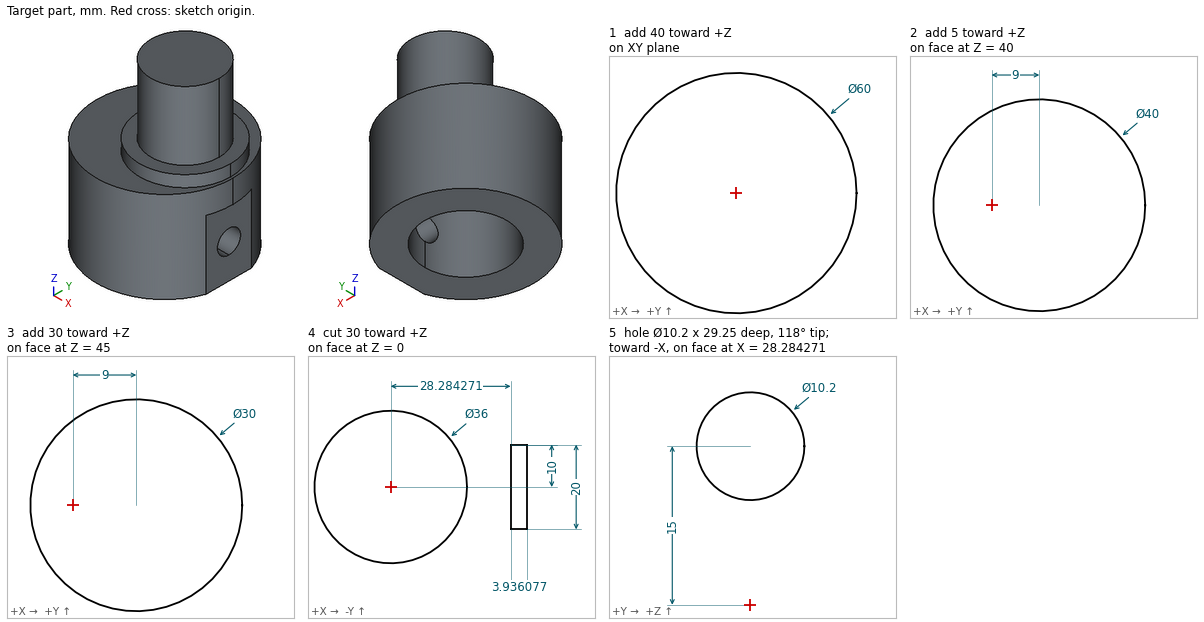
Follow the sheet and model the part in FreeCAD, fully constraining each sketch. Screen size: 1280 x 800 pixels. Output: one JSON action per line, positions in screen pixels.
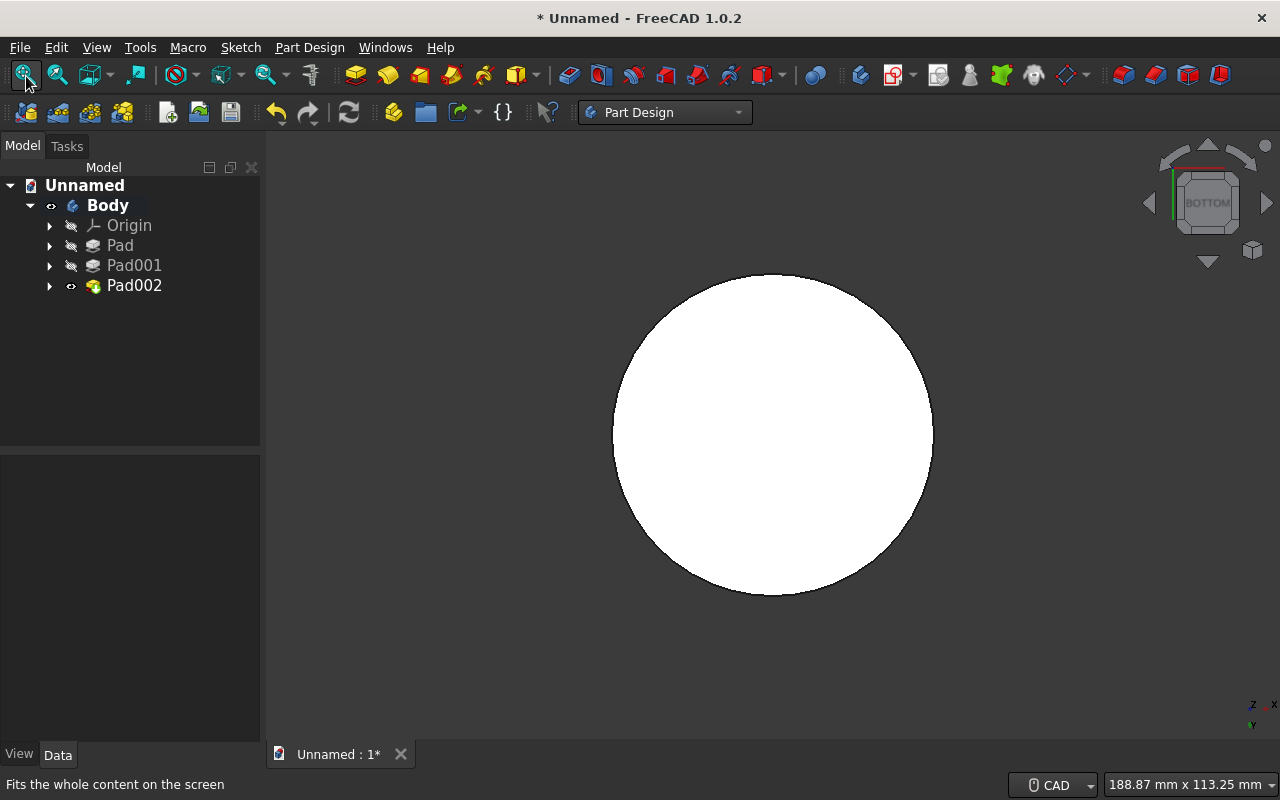
{"action": "left_click", "coordinate": [773, 434]}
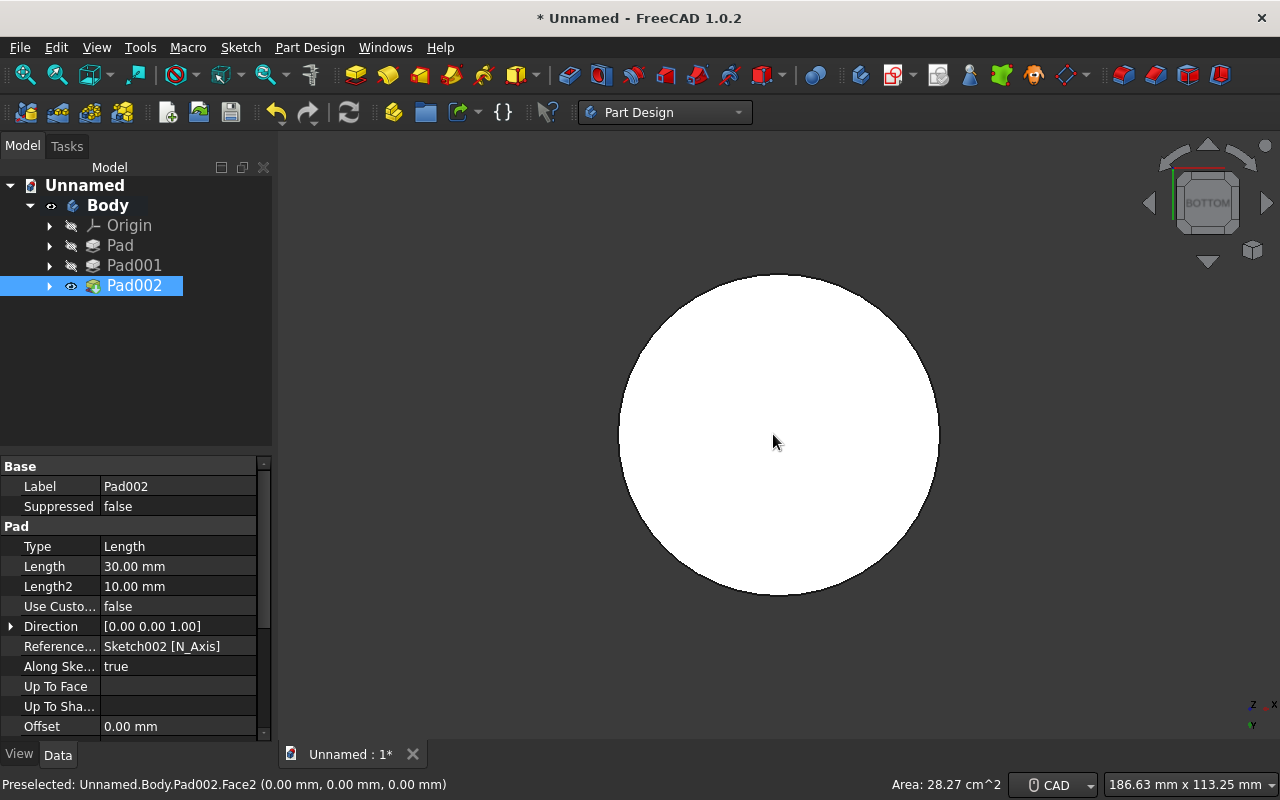
{"action": "left_click", "coordinate": [894, 76]}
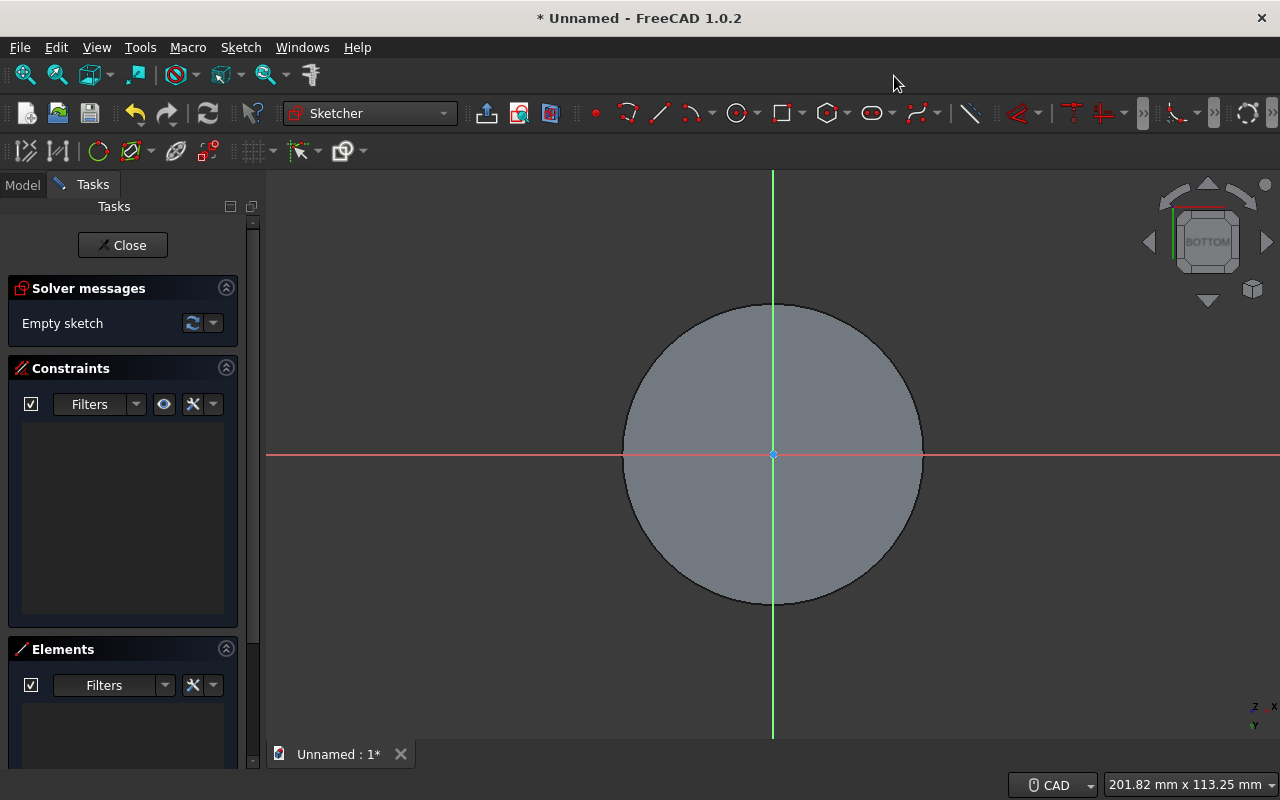
{"action": "scroll", "coordinate": [935, 454], "scroll_direction": "up", "scroll_amount": 3}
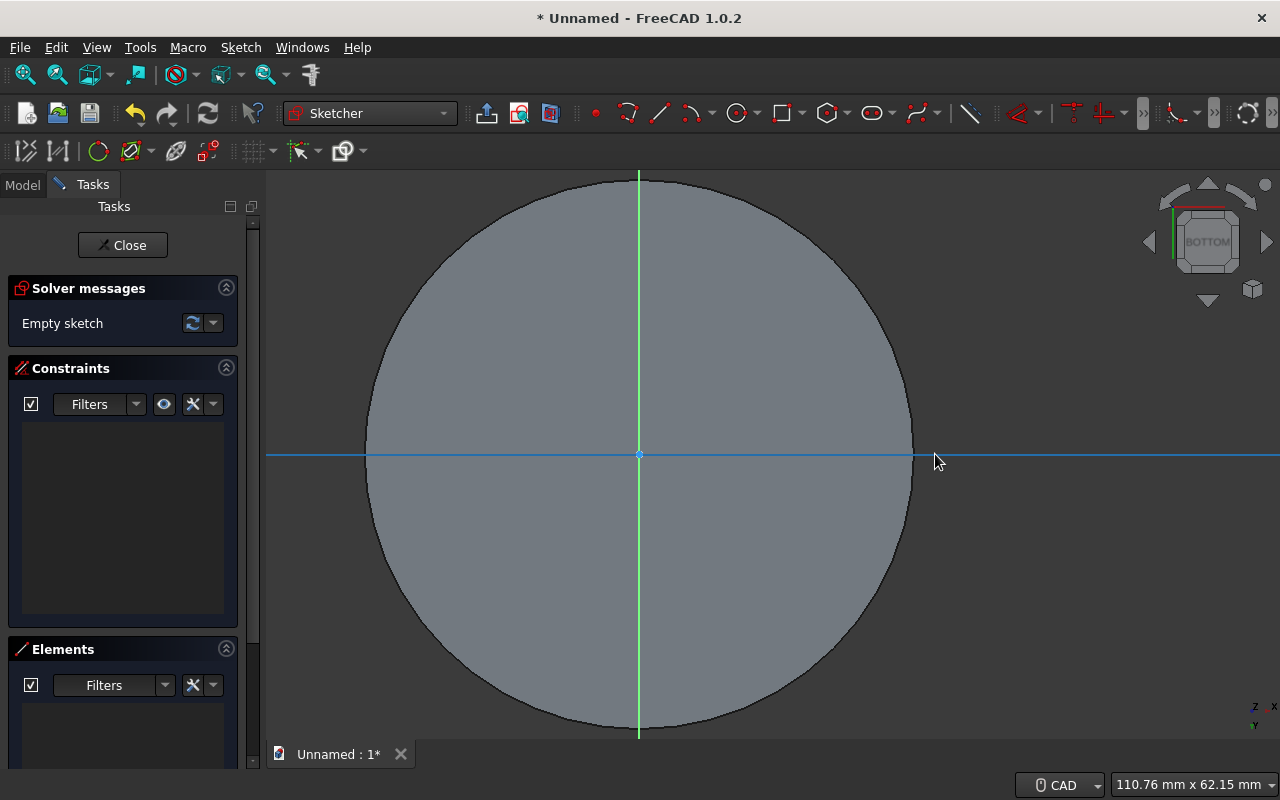
{"action": "left_click", "coordinate": [782, 114]}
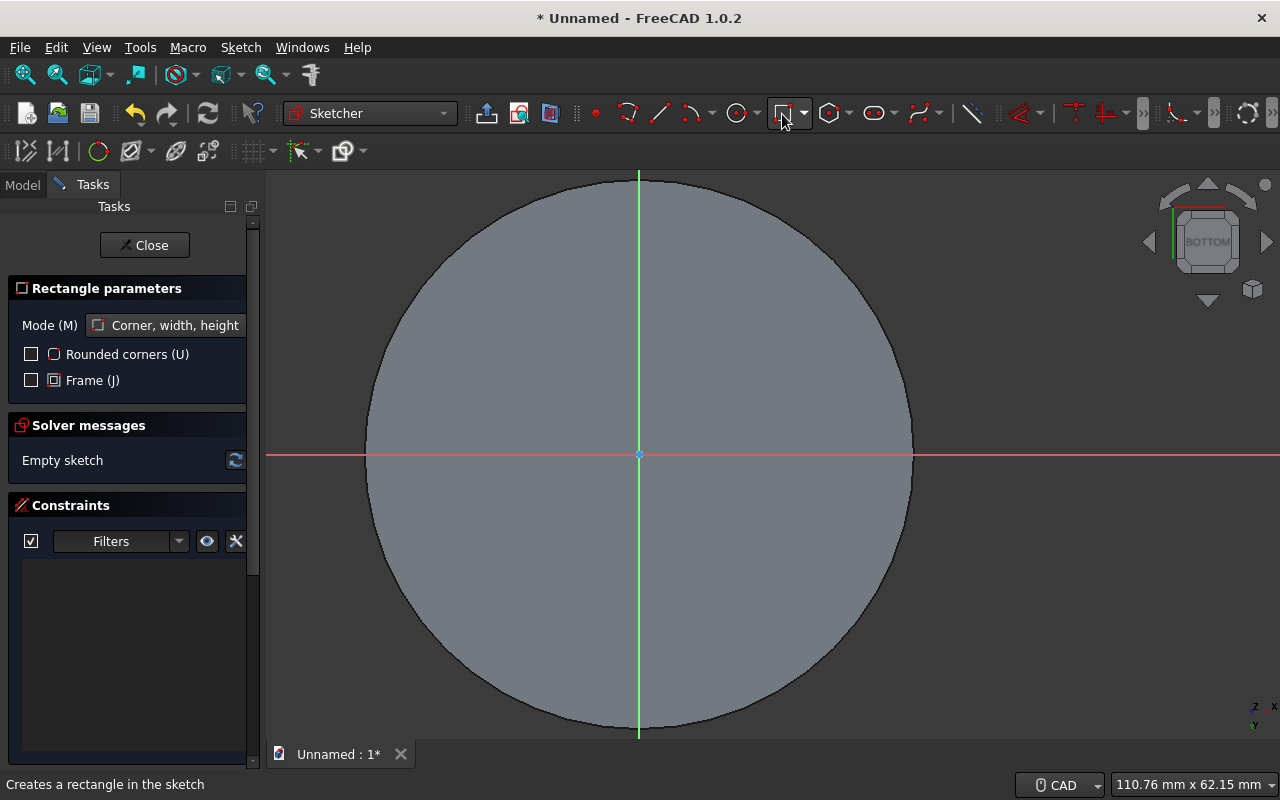
{"action": "left_click", "coordinate": [898, 363]}
{"action": "mouse_move", "coordinate": [934, 546]}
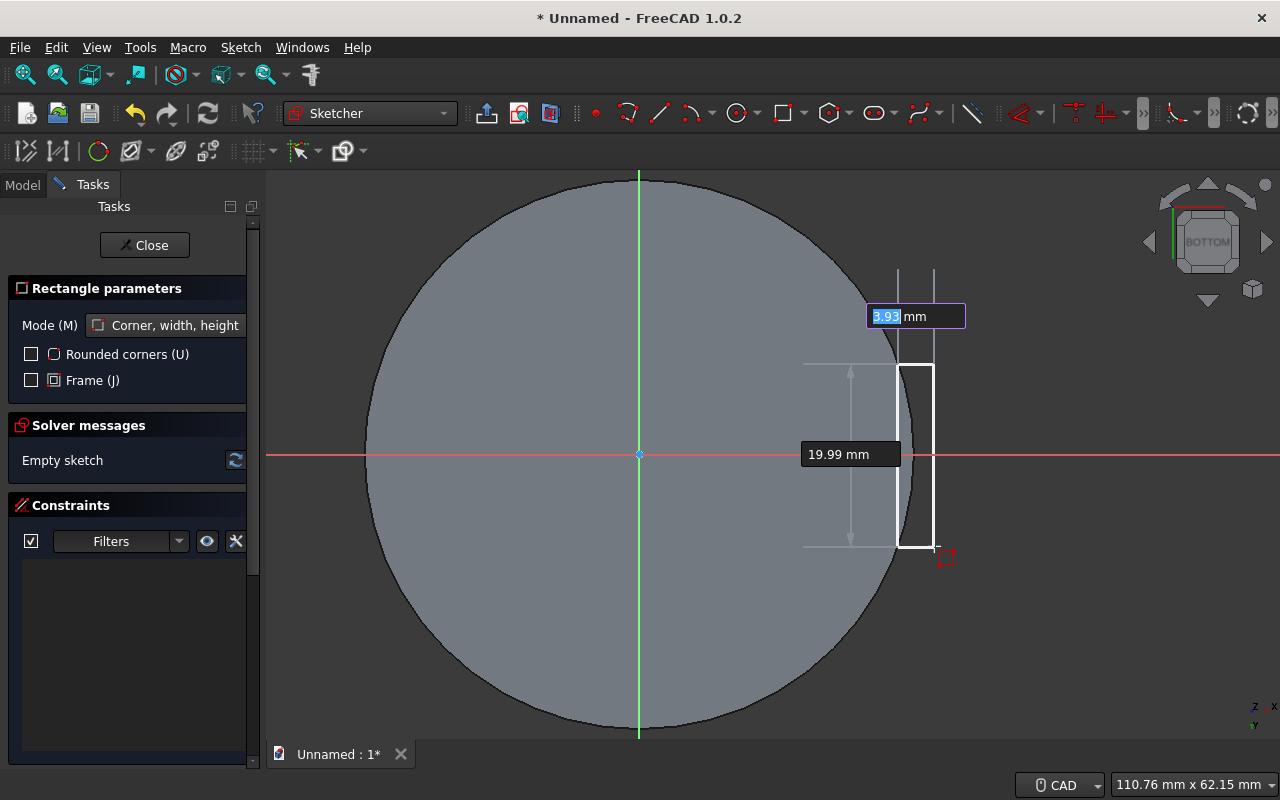
{"action": "type", "text": "3.936077"}
{"action": "key", "text": "Tab"}
{"action": "type", "text": "20"}
{"action": "key", "text": "Return"}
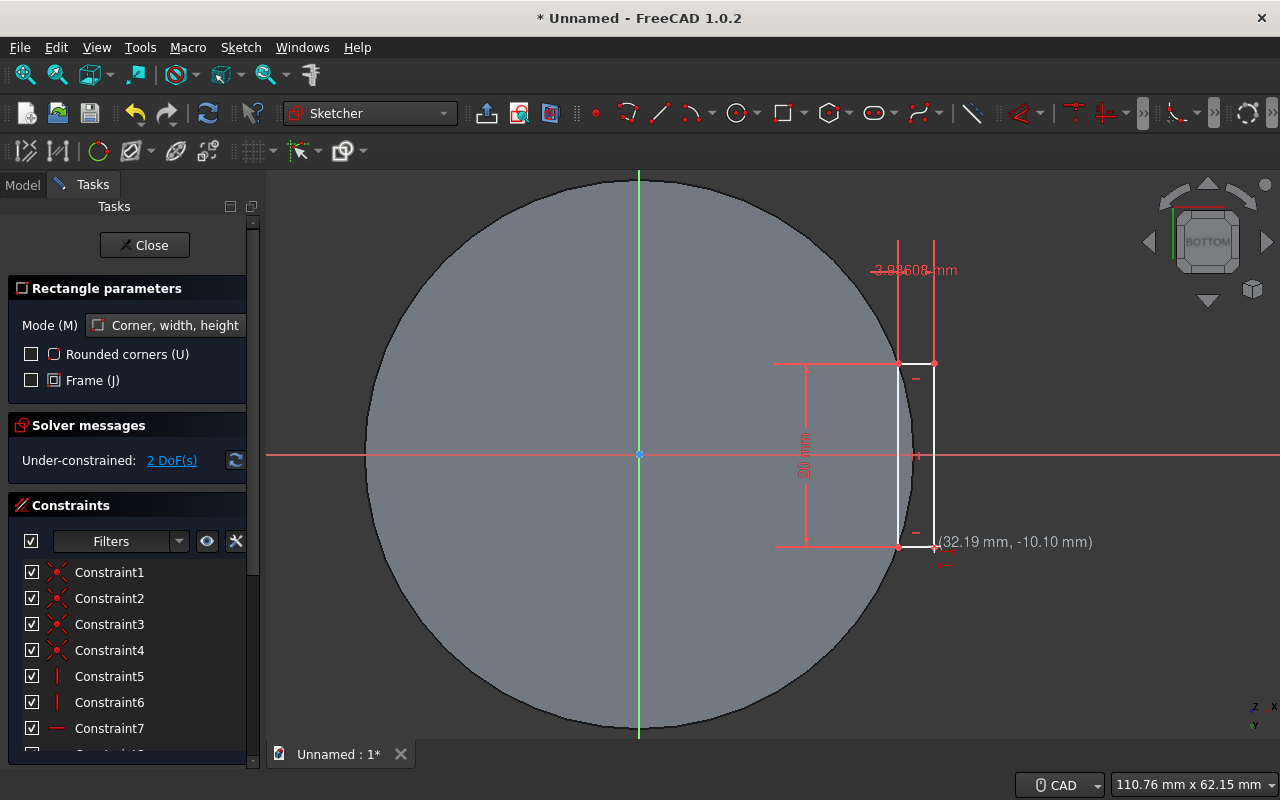
{"action": "left_click", "coordinate": [738, 114]}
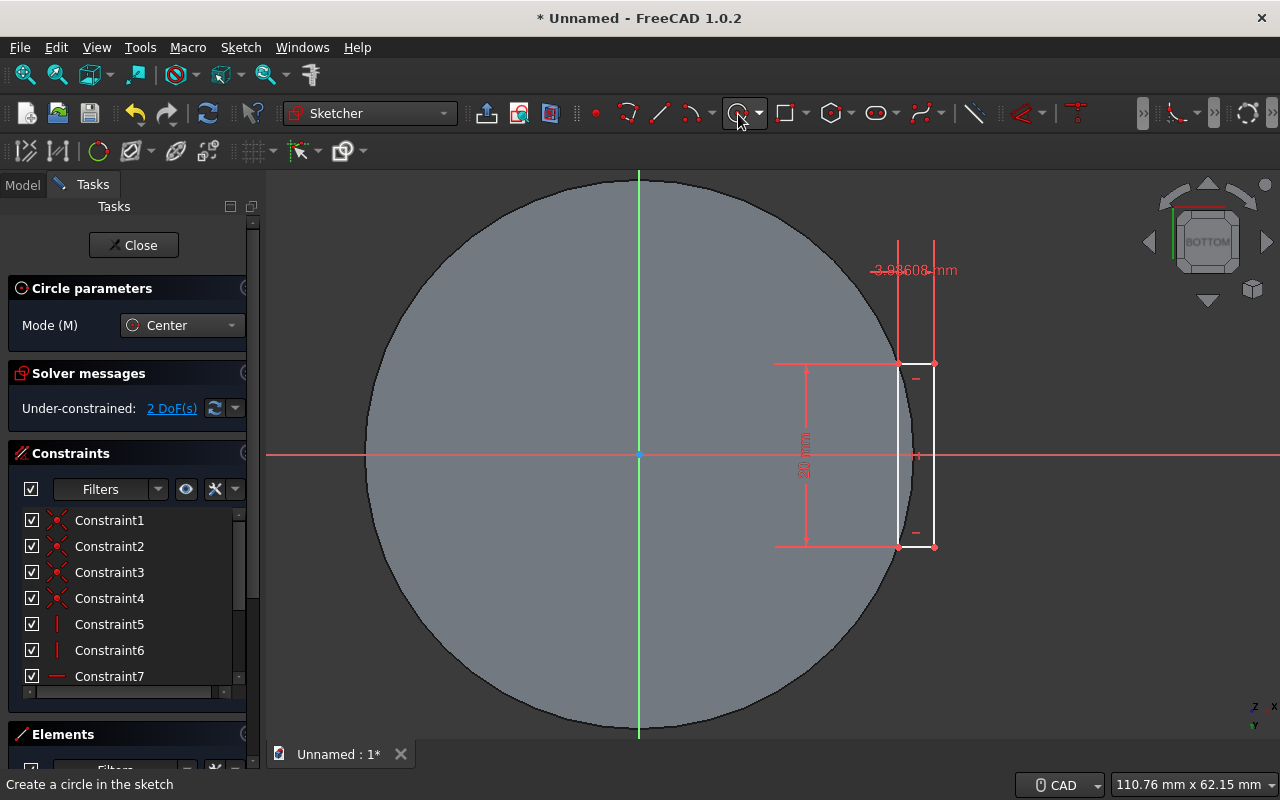
{"action": "left_click", "coordinate": [639, 454]}
{"action": "mouse_move", "coordinate": [756, 338]}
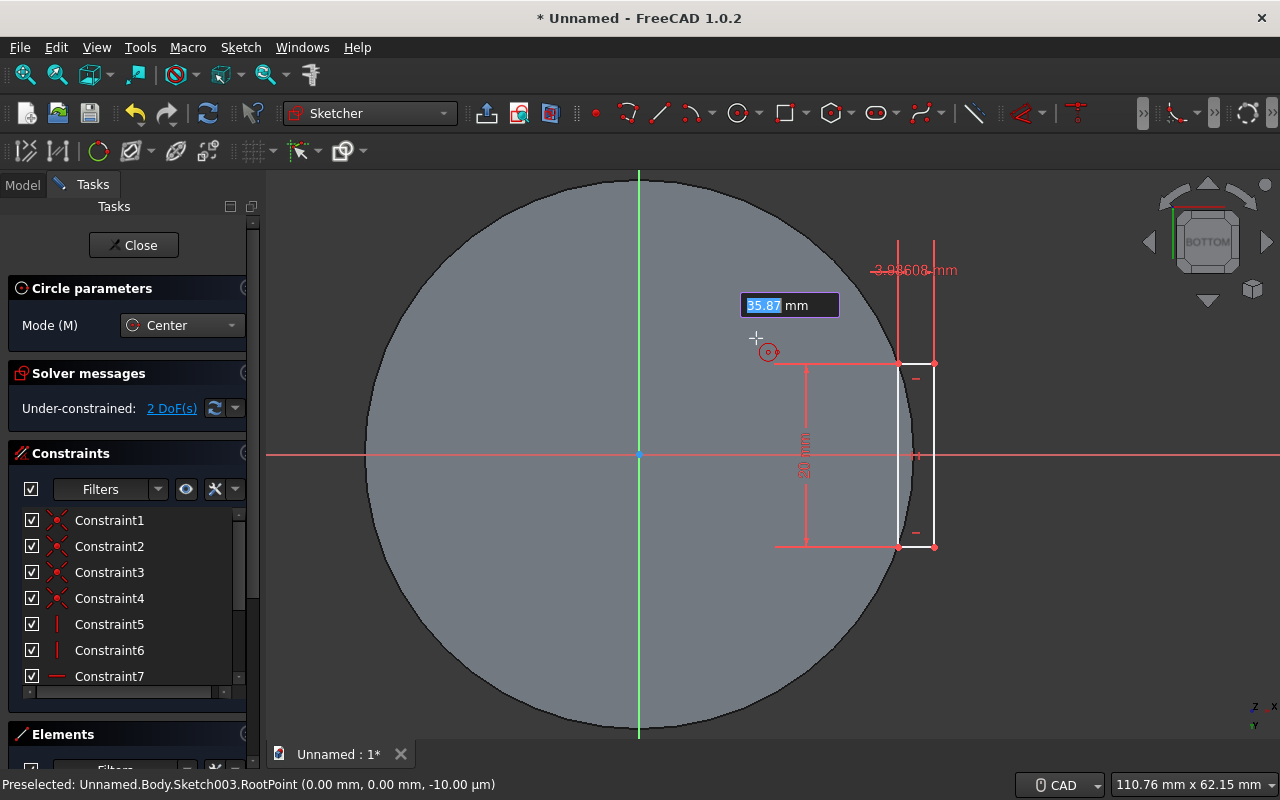
{"action": "type", "text": "36"}
{"action": "key", "text": "Return"}
{"action": "key", "text": "Escape"}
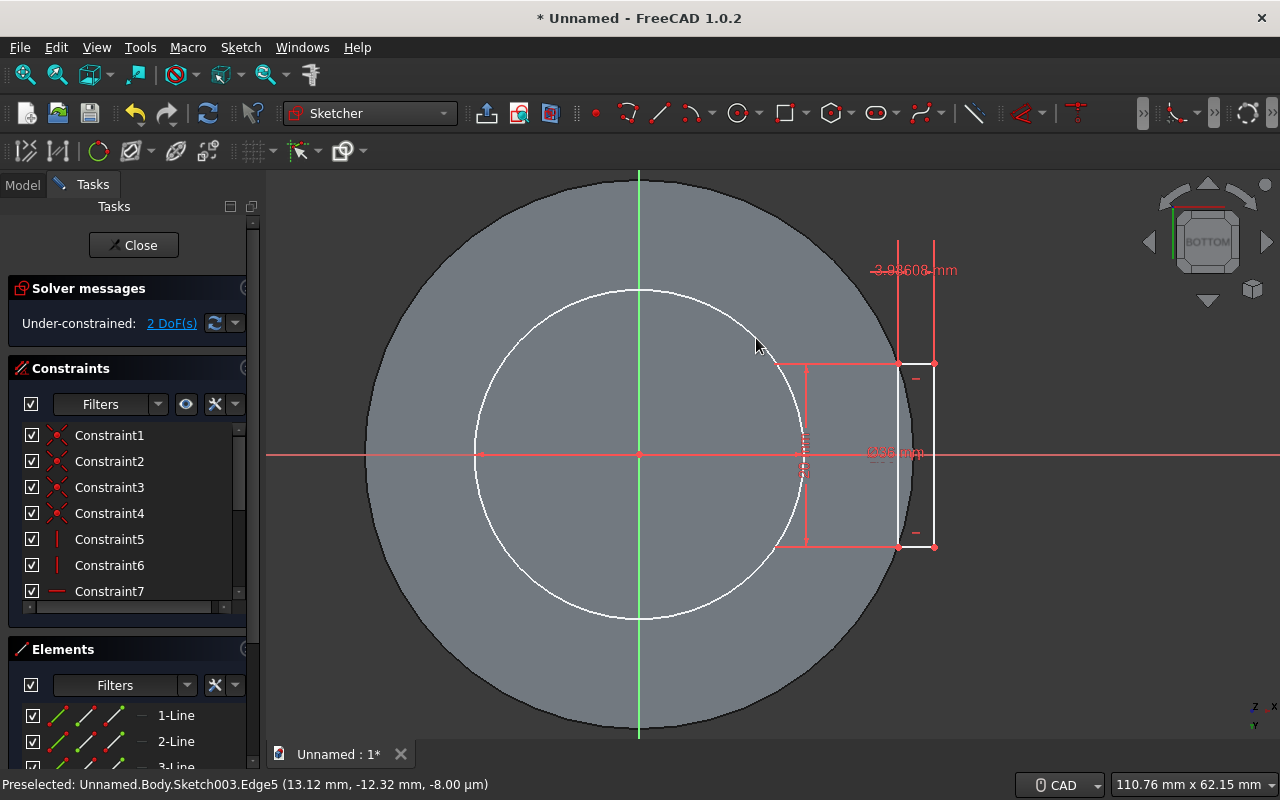
{"action": "key", "text": "d"}